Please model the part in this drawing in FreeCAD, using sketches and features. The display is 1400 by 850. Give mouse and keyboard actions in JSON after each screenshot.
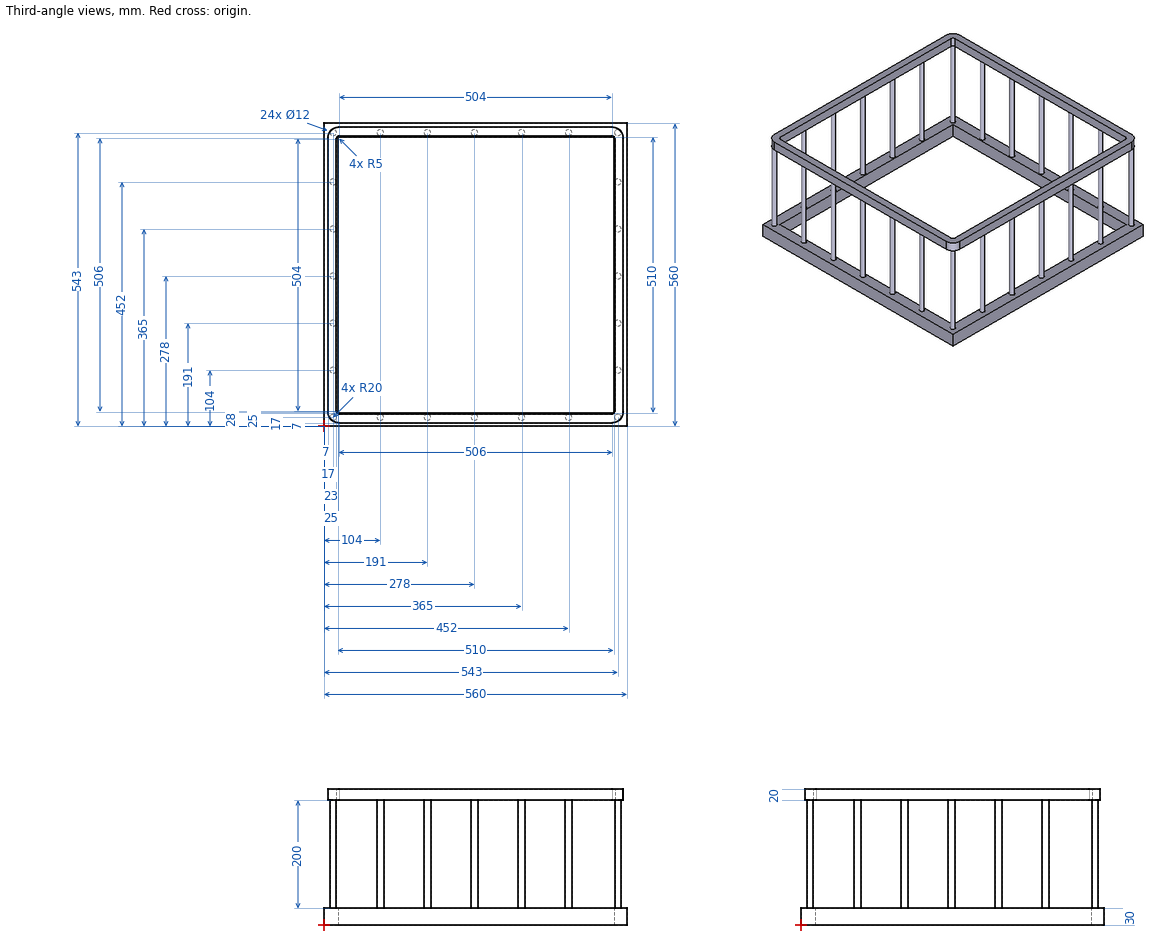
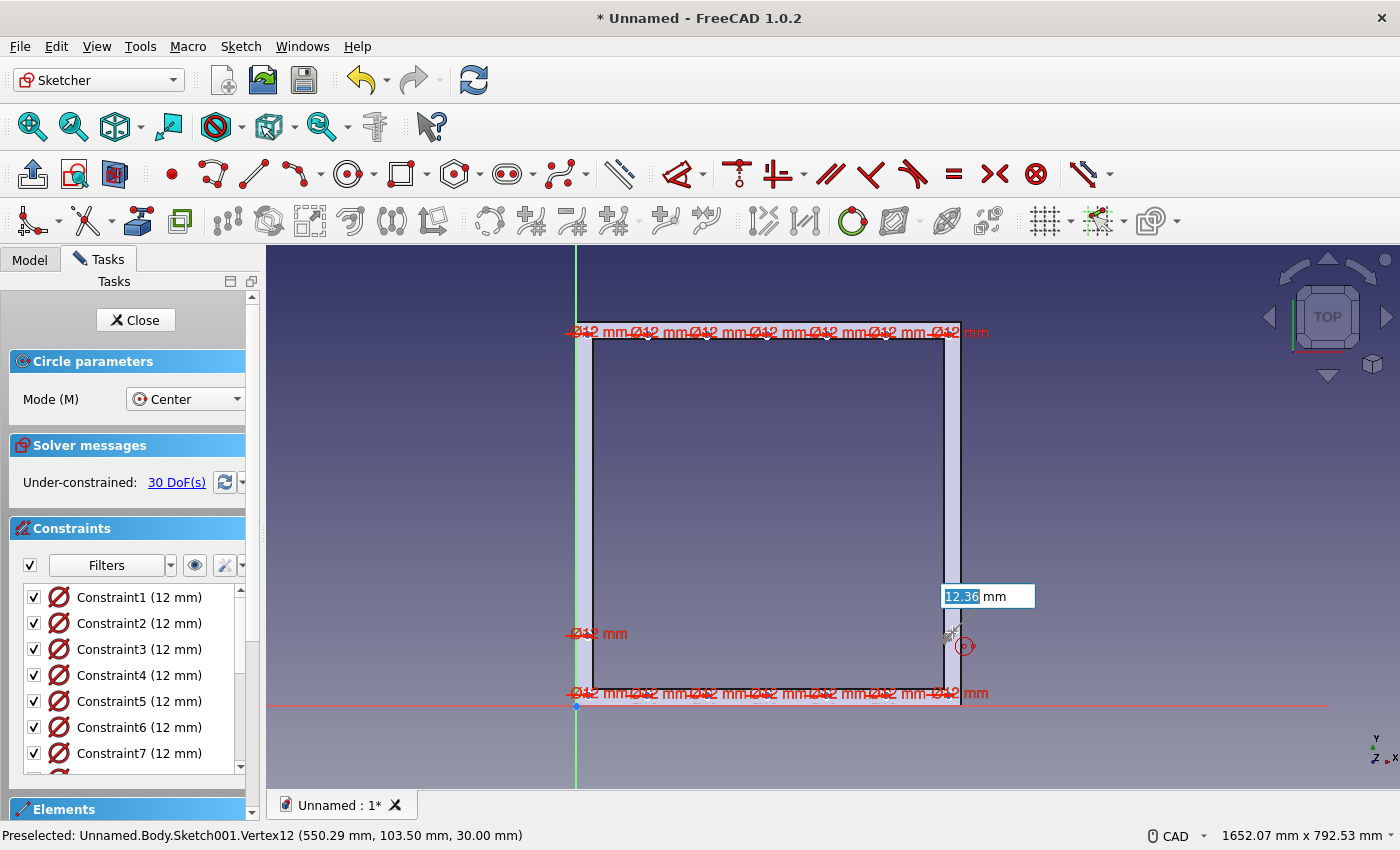
{"action": "type", "text": "12"}
{"action": "key", "text": "Return"}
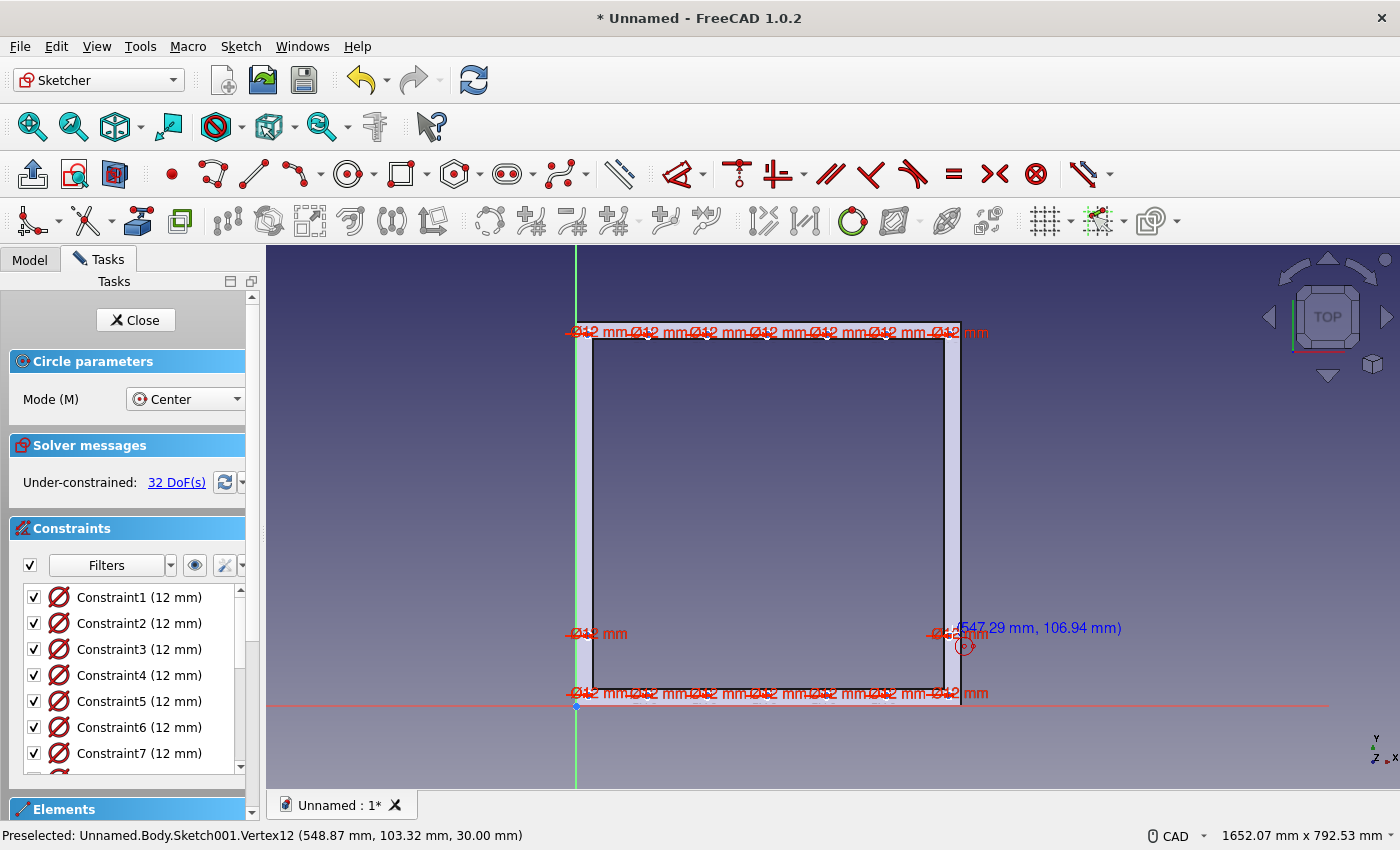
{"action": "scroll", "coordinate": [588, 575], "scroll_direction": "up", "scroll_amount": 9}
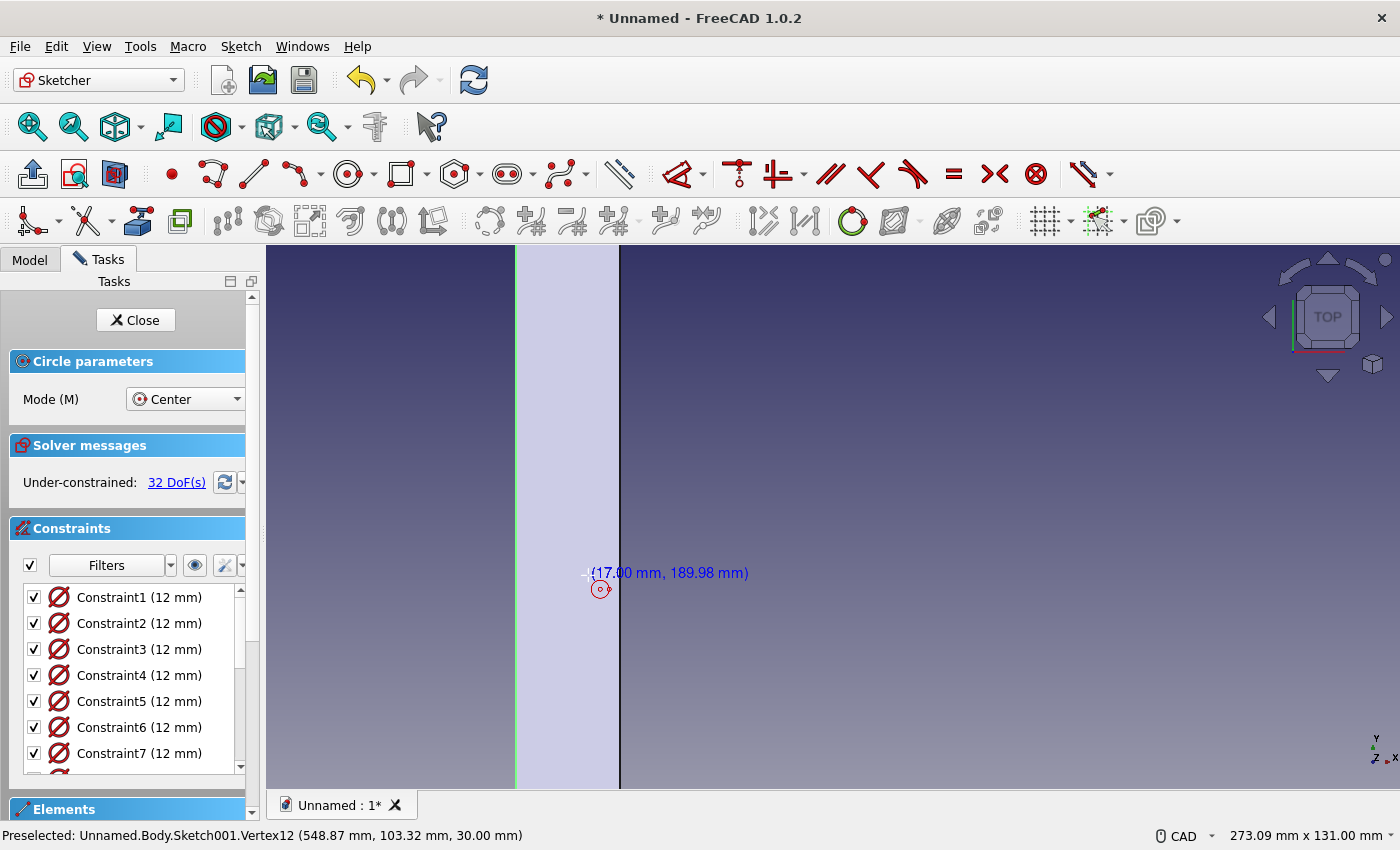
{"action": "scroll", "coordinate": [588, 574], "scroll_direction": "down", "scroll_amount": 9}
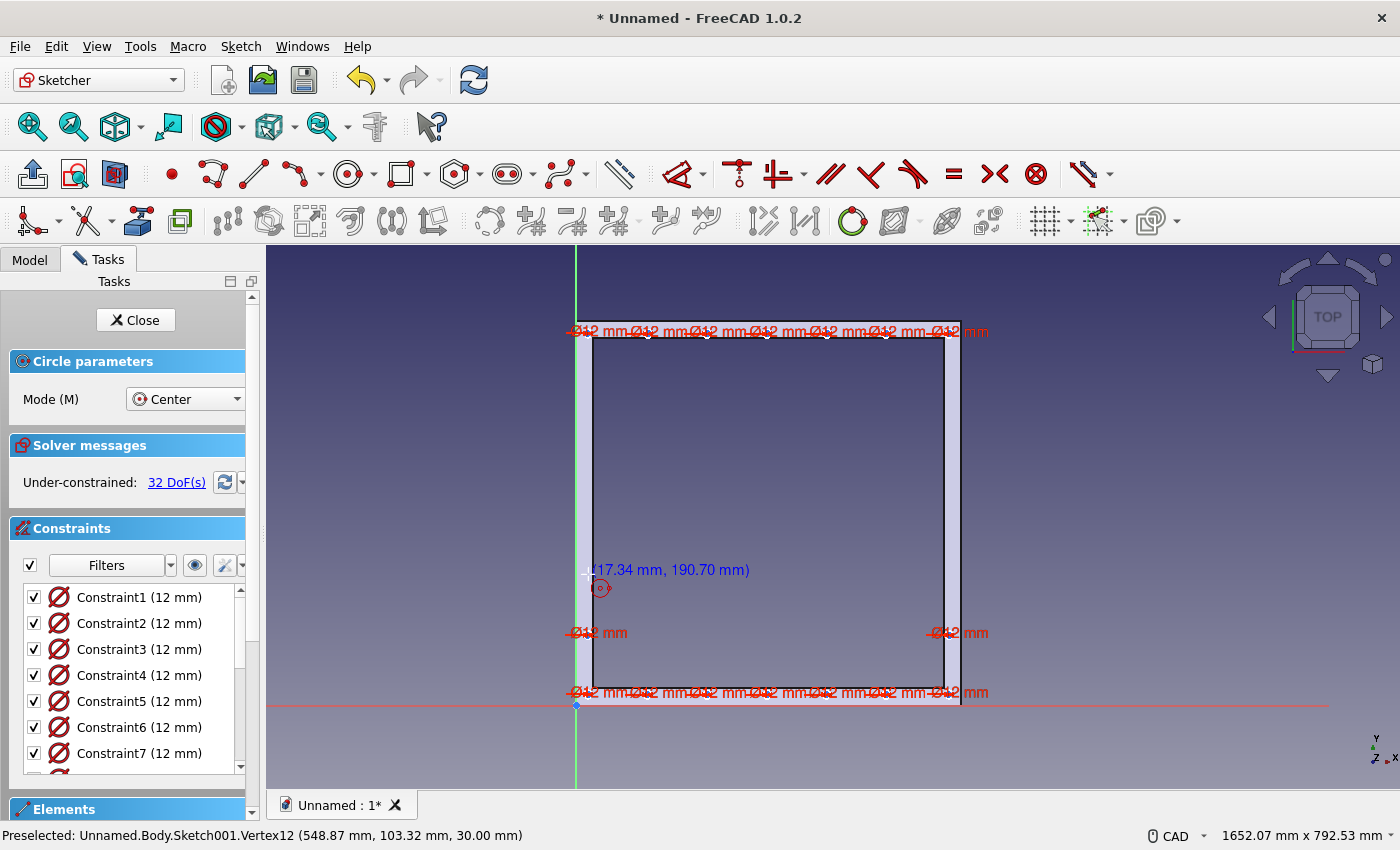
{"action": "scroll", "coordinate": [588, 574], "scroll_direction": "up", "scroll_amount": 2}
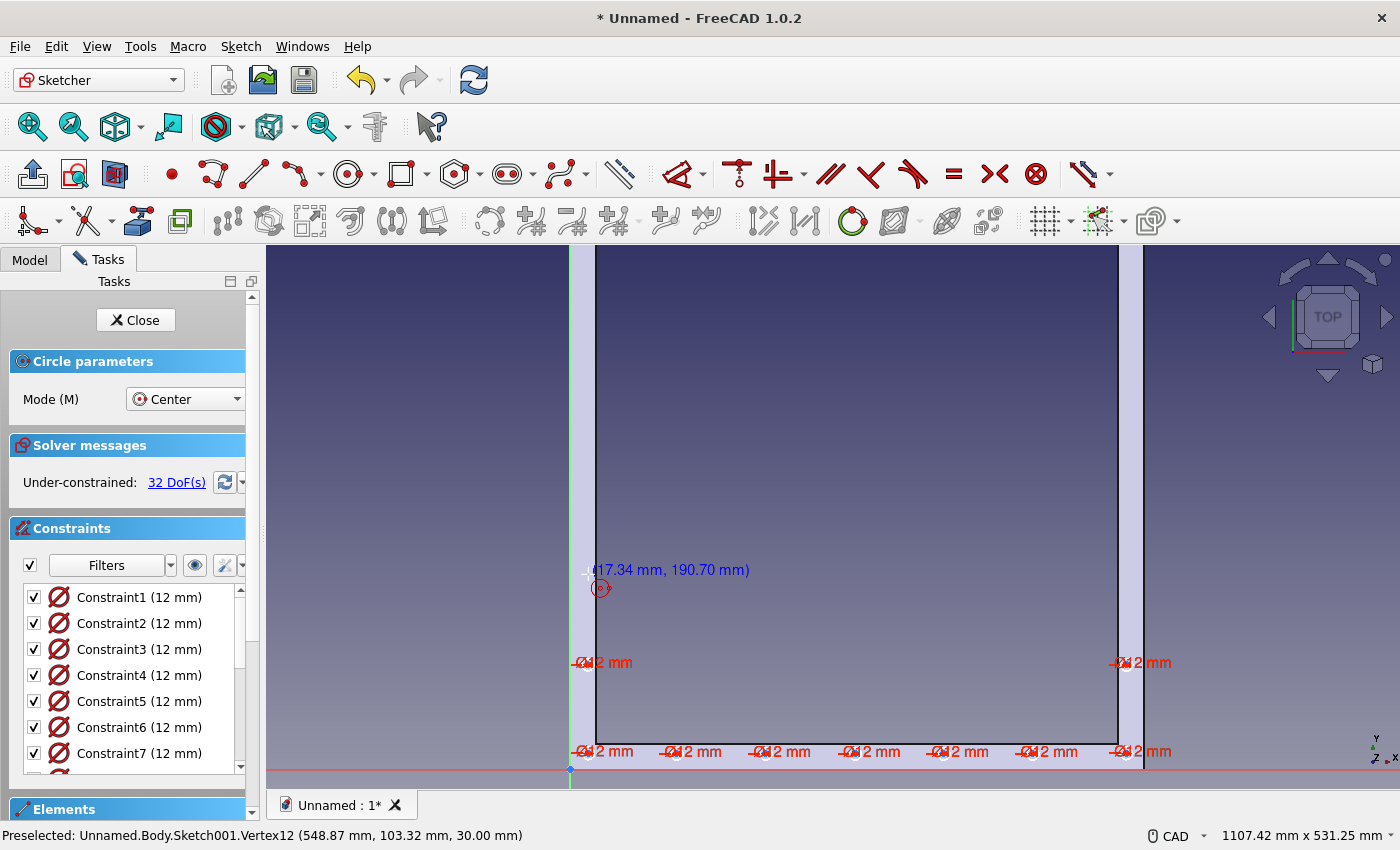
{"action": "left_click", "coordinate": [588, 574]}
{"action": "mouse_move", "coordinate": [592, 570]}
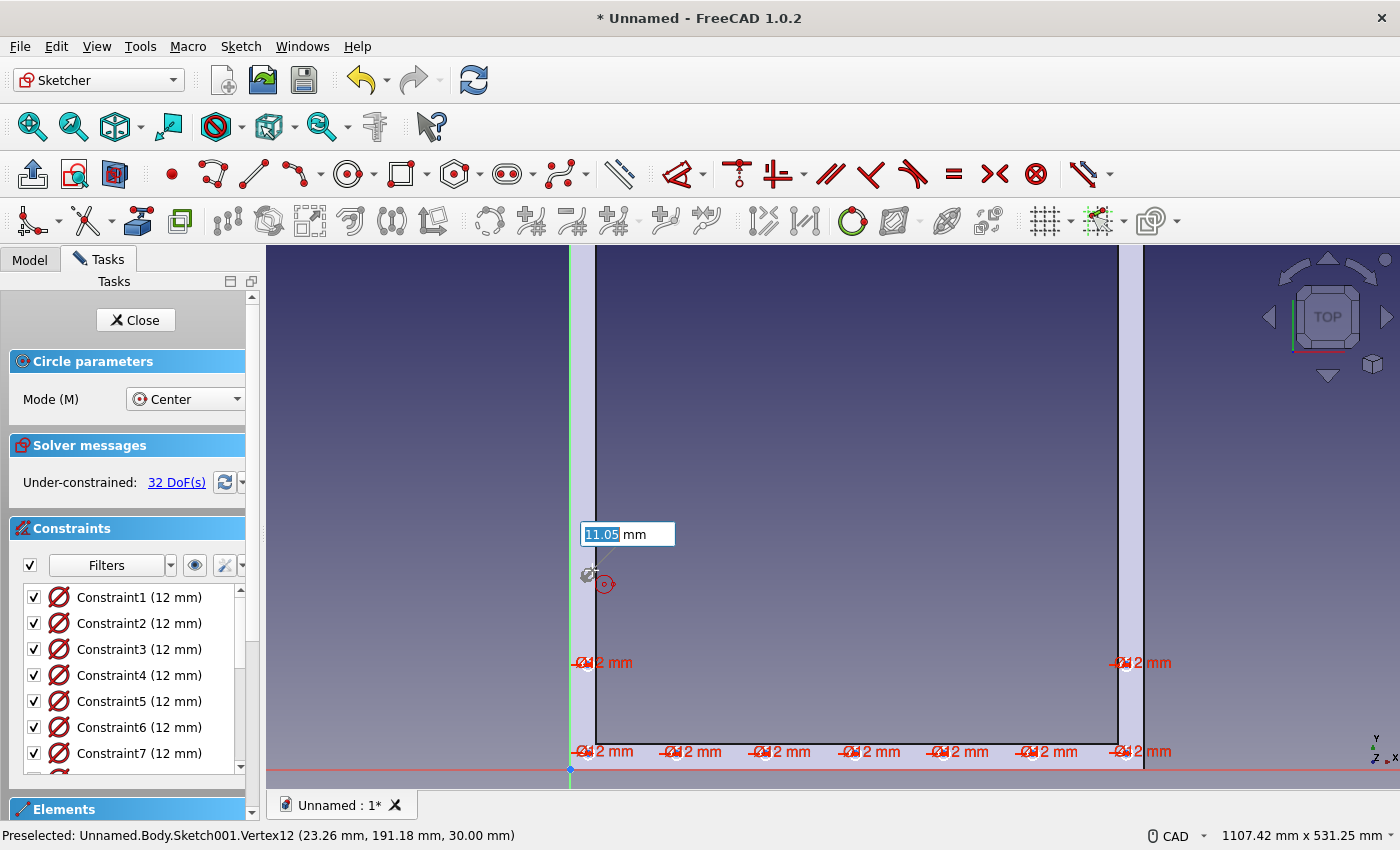
{"action": "type", "text": "12"}
{"action": "key", "text": "Return"}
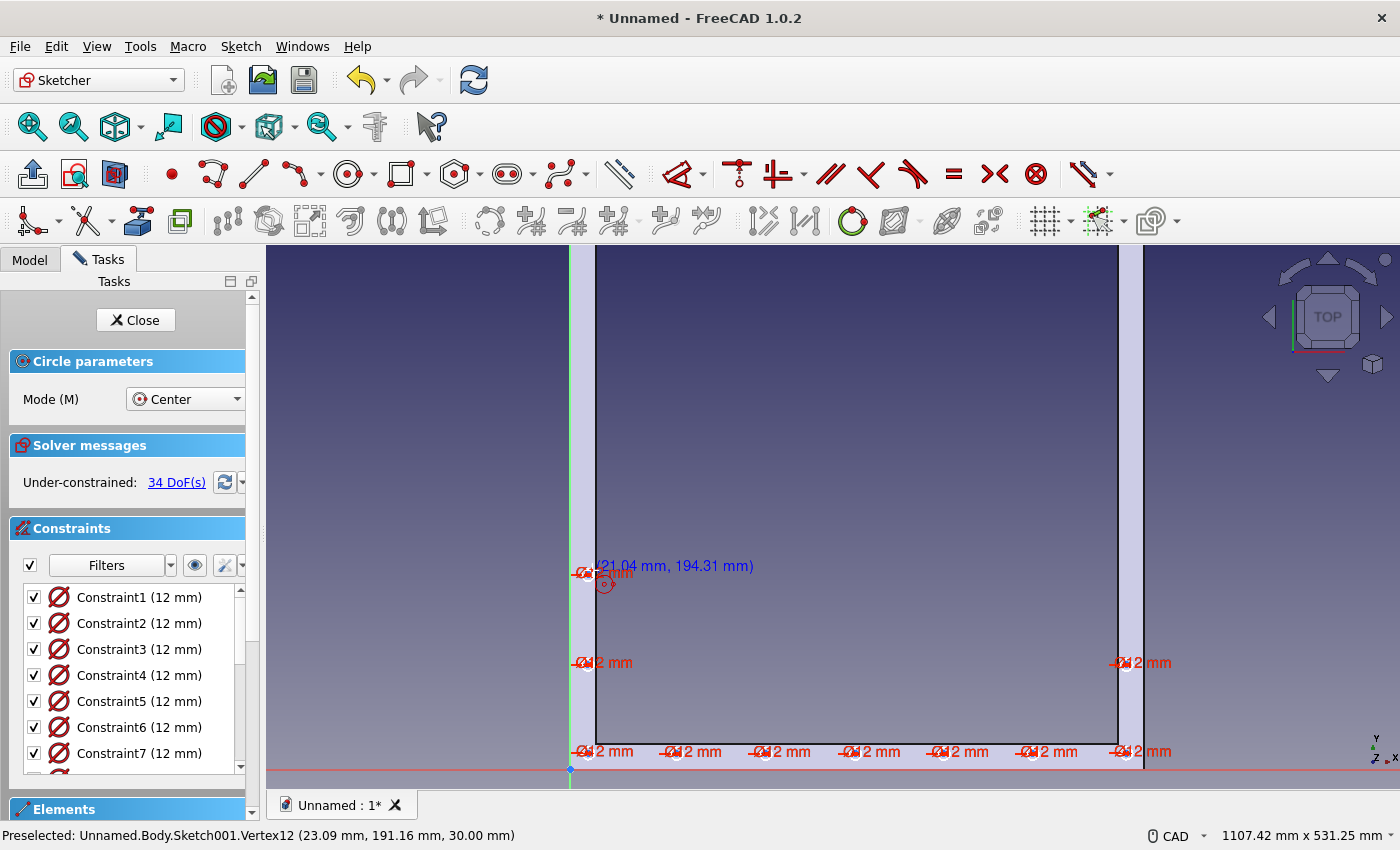
{"action": "scroll", "coordinate": [1126, 574], "scroll_direction": "up", "scroll_amount": 7}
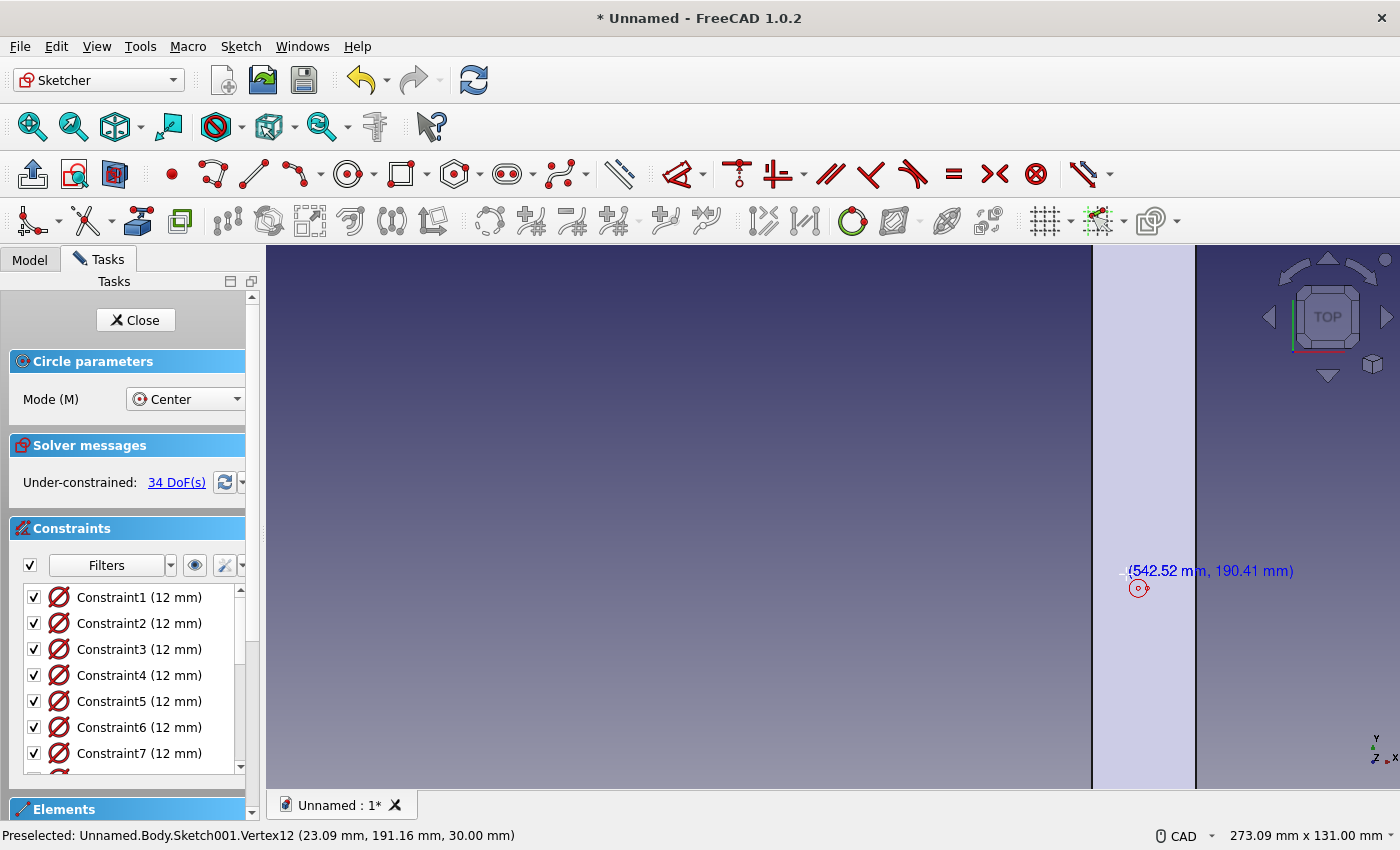
{"action": "scroll", "coordinate": [914, 574], "scroll_direction": "down", "scroll_amount": 9}